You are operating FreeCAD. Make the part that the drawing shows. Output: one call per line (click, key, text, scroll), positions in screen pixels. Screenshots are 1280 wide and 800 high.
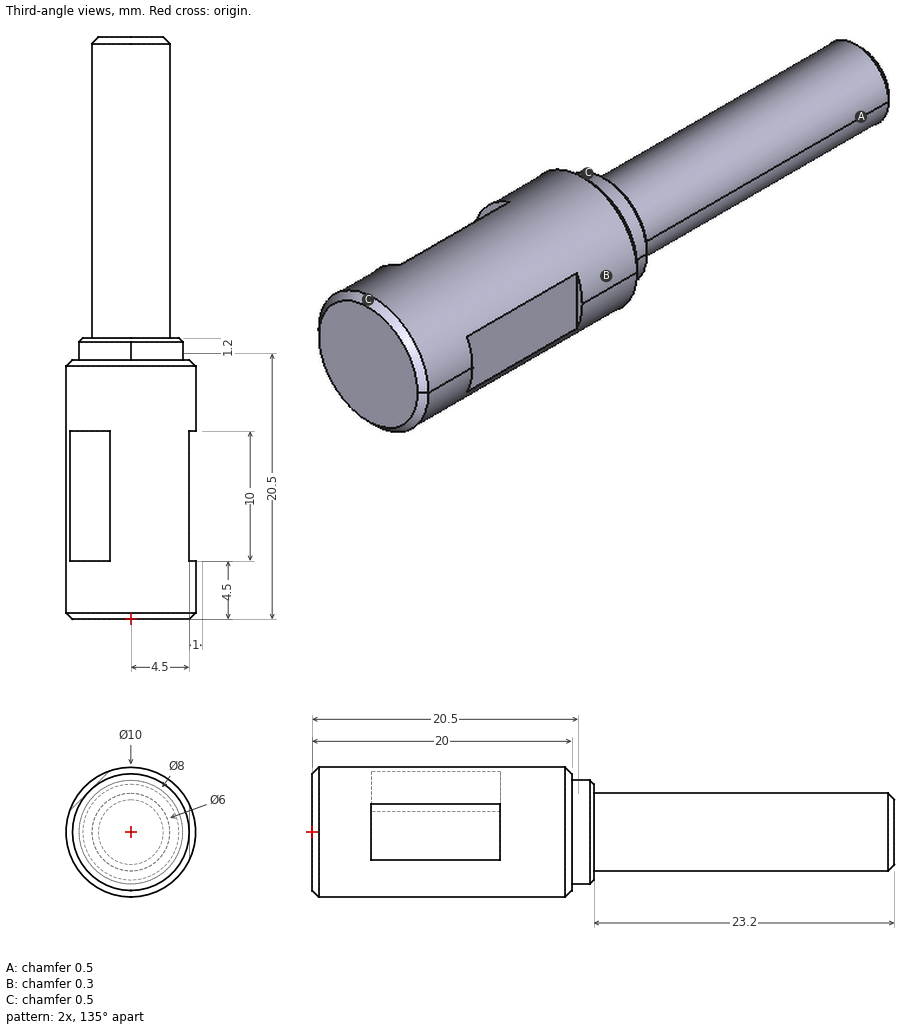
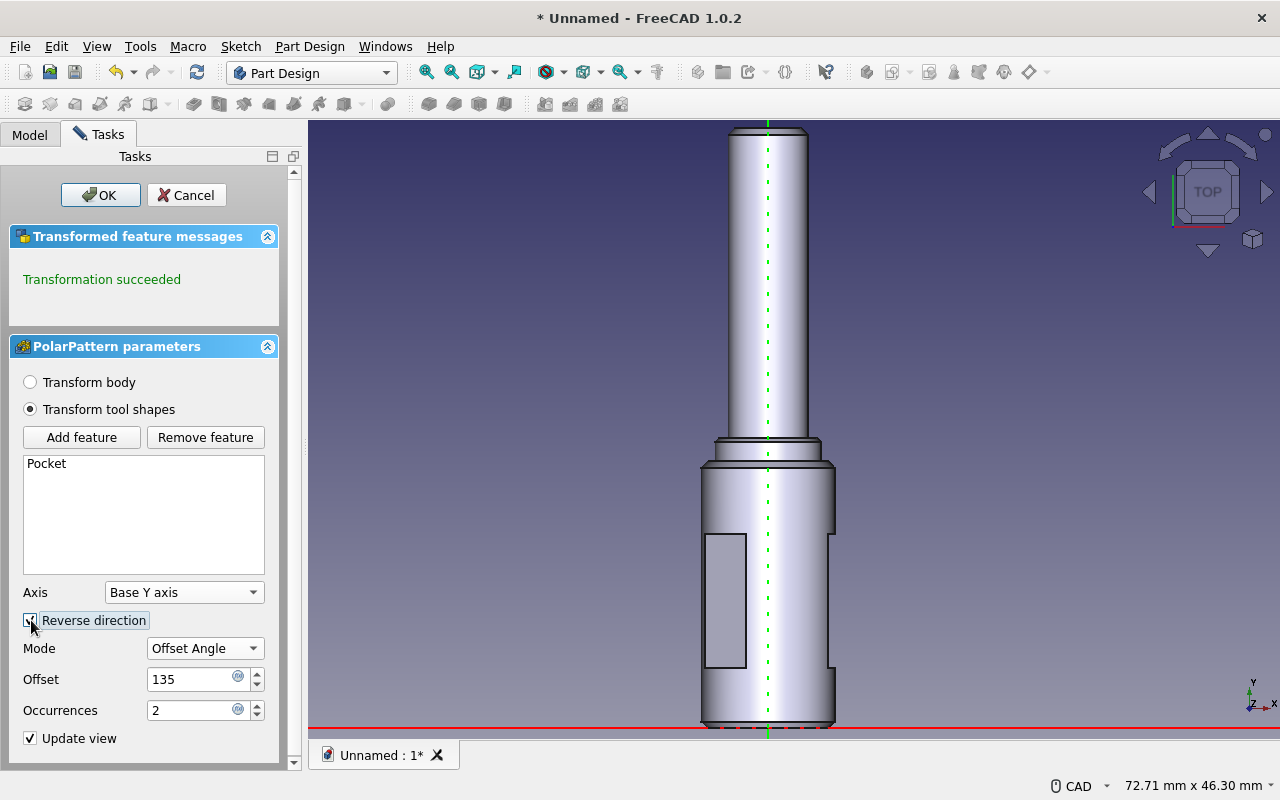
click(101, 195)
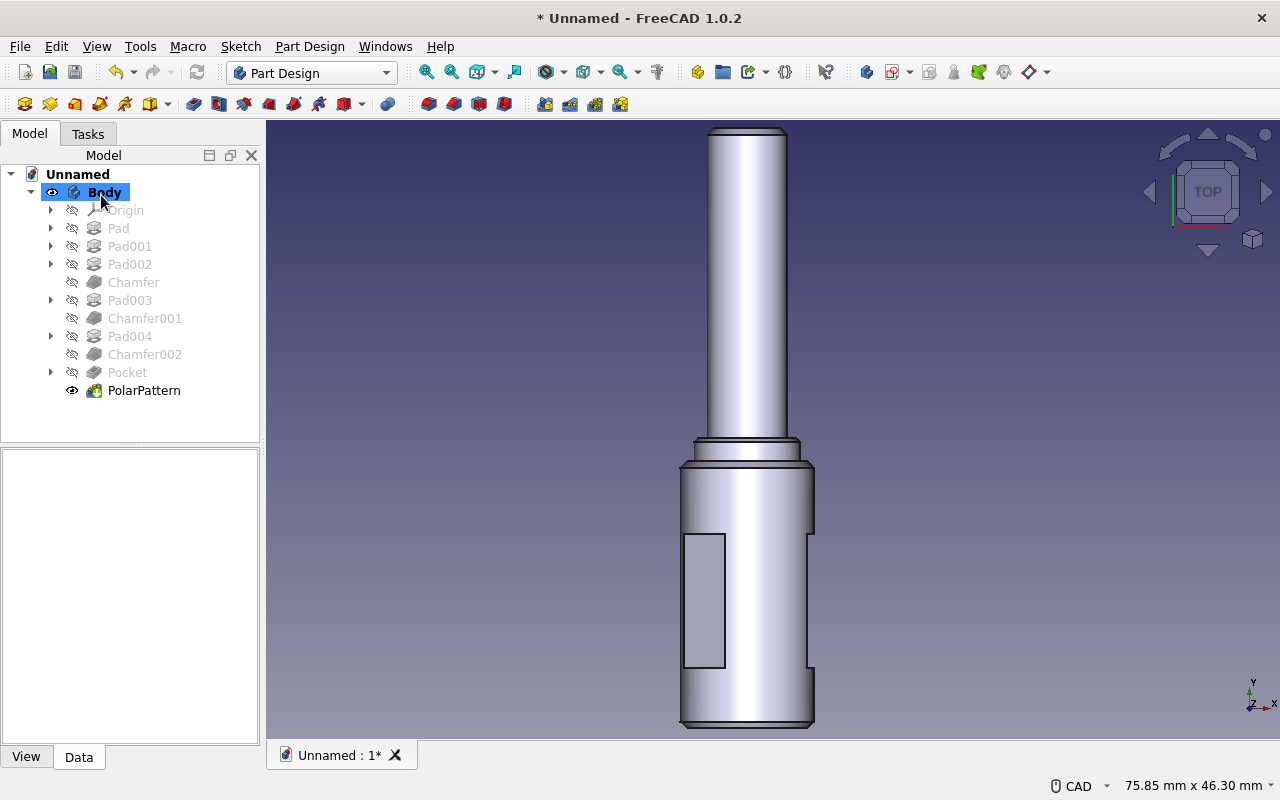
key(0)